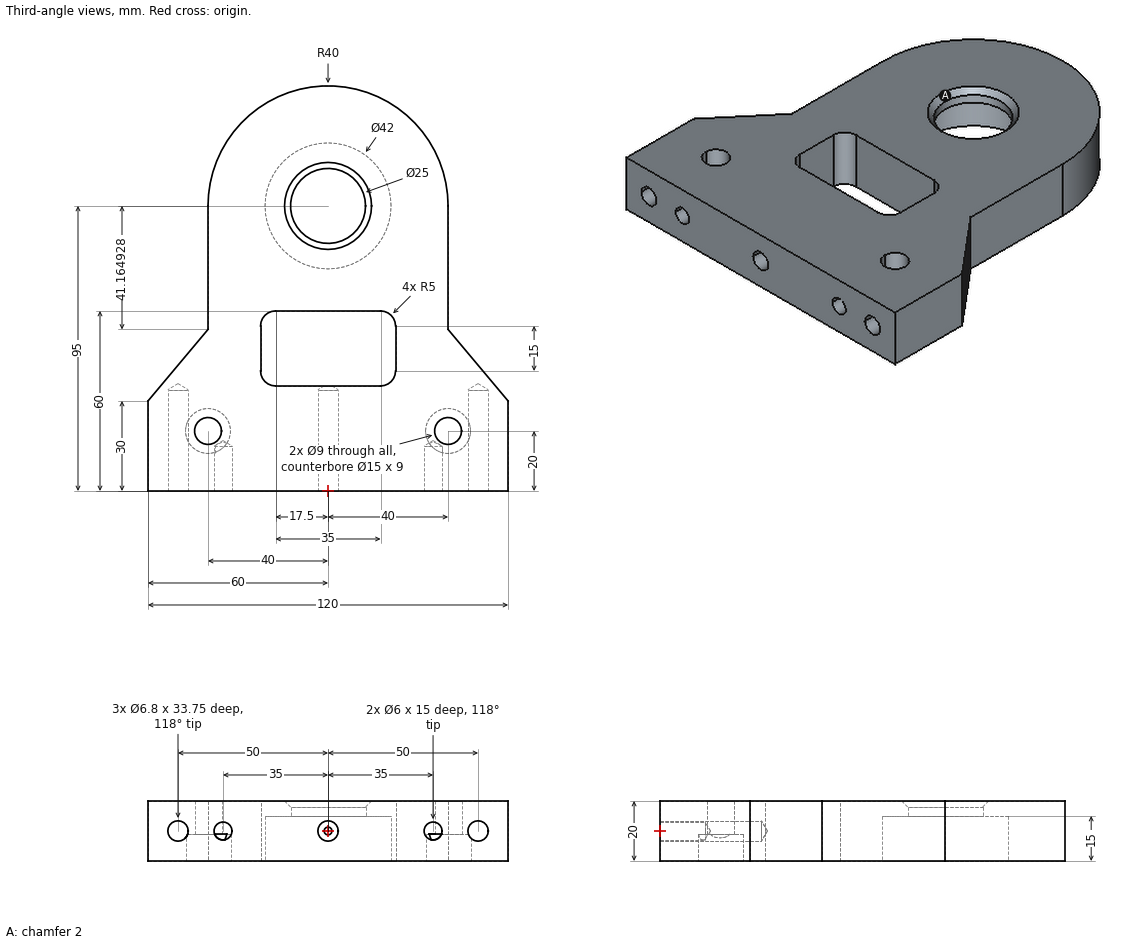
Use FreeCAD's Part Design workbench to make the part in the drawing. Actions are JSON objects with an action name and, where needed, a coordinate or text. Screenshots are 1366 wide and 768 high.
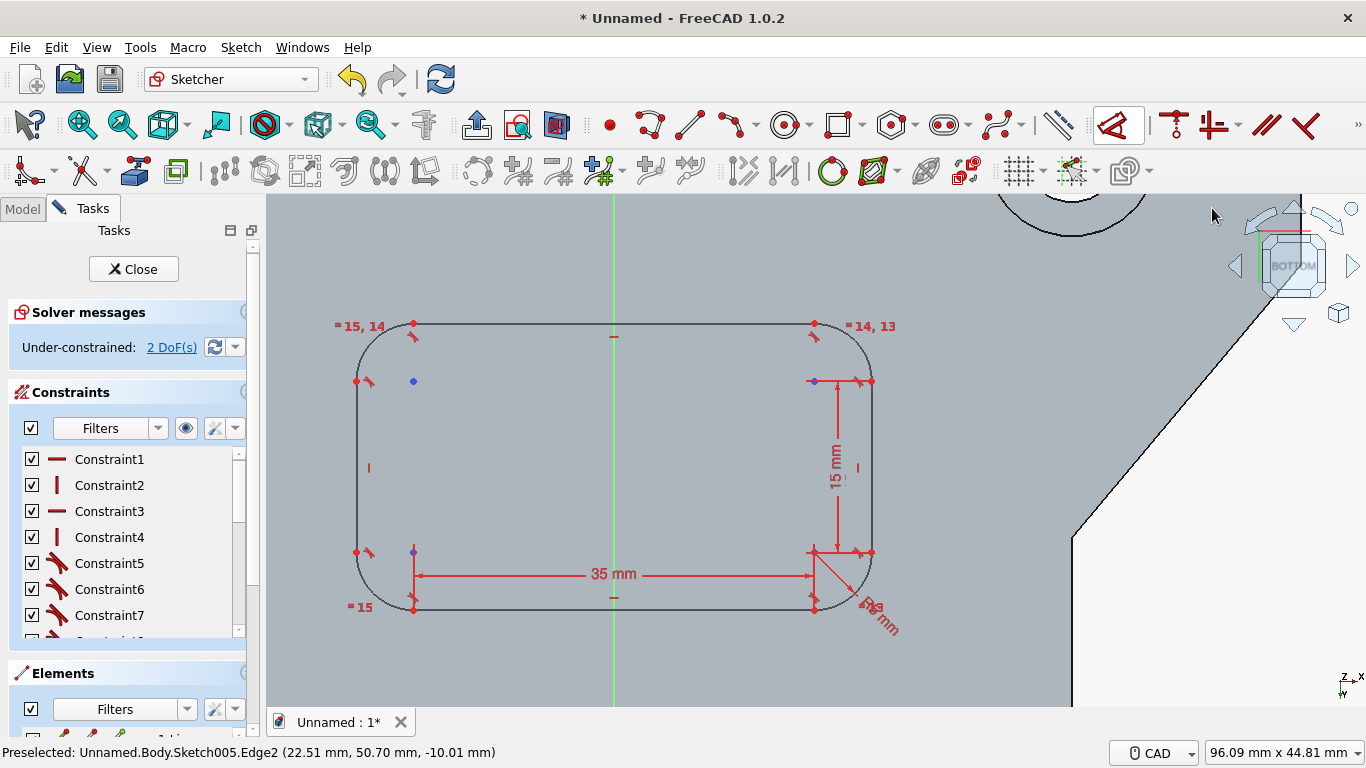
{"action": "left_click", "coordinate": [414, 610]}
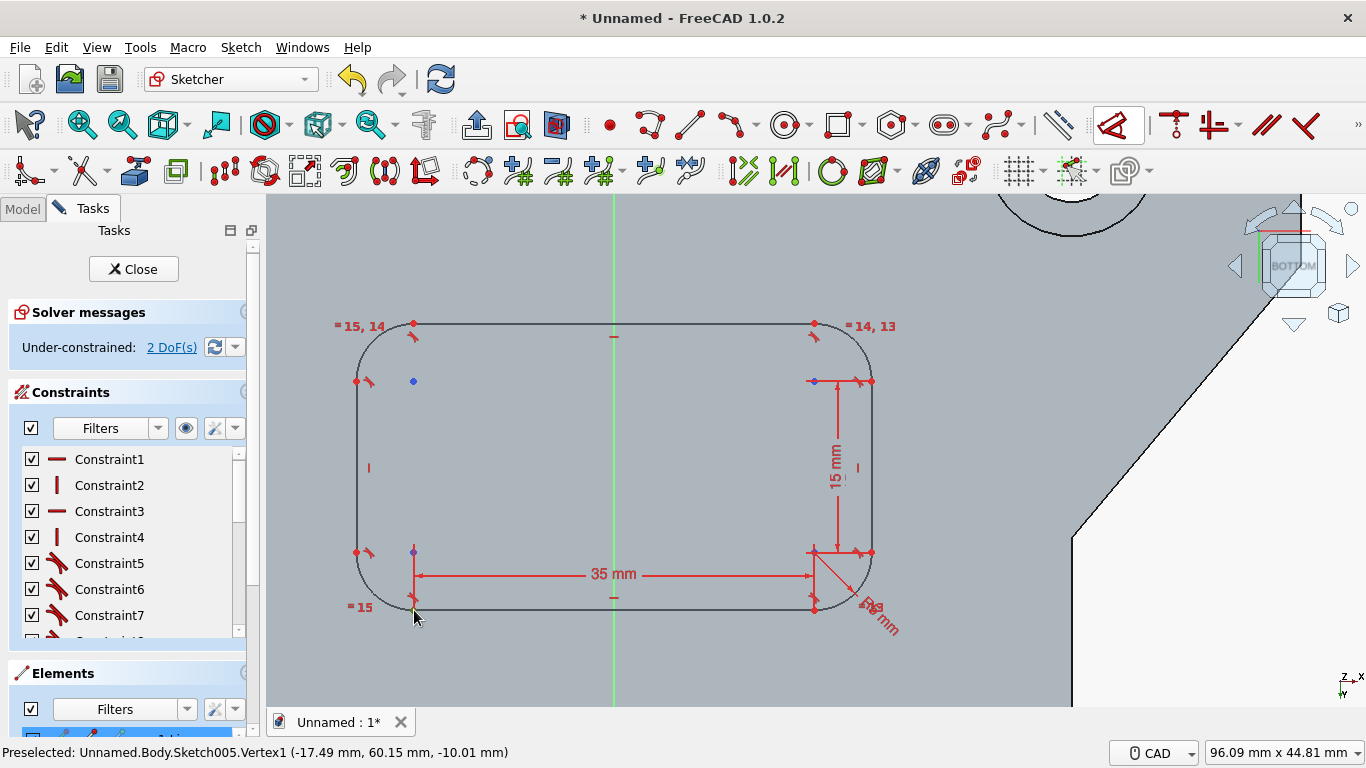
{"action": "left_click", "coordinate": [1138, 126]}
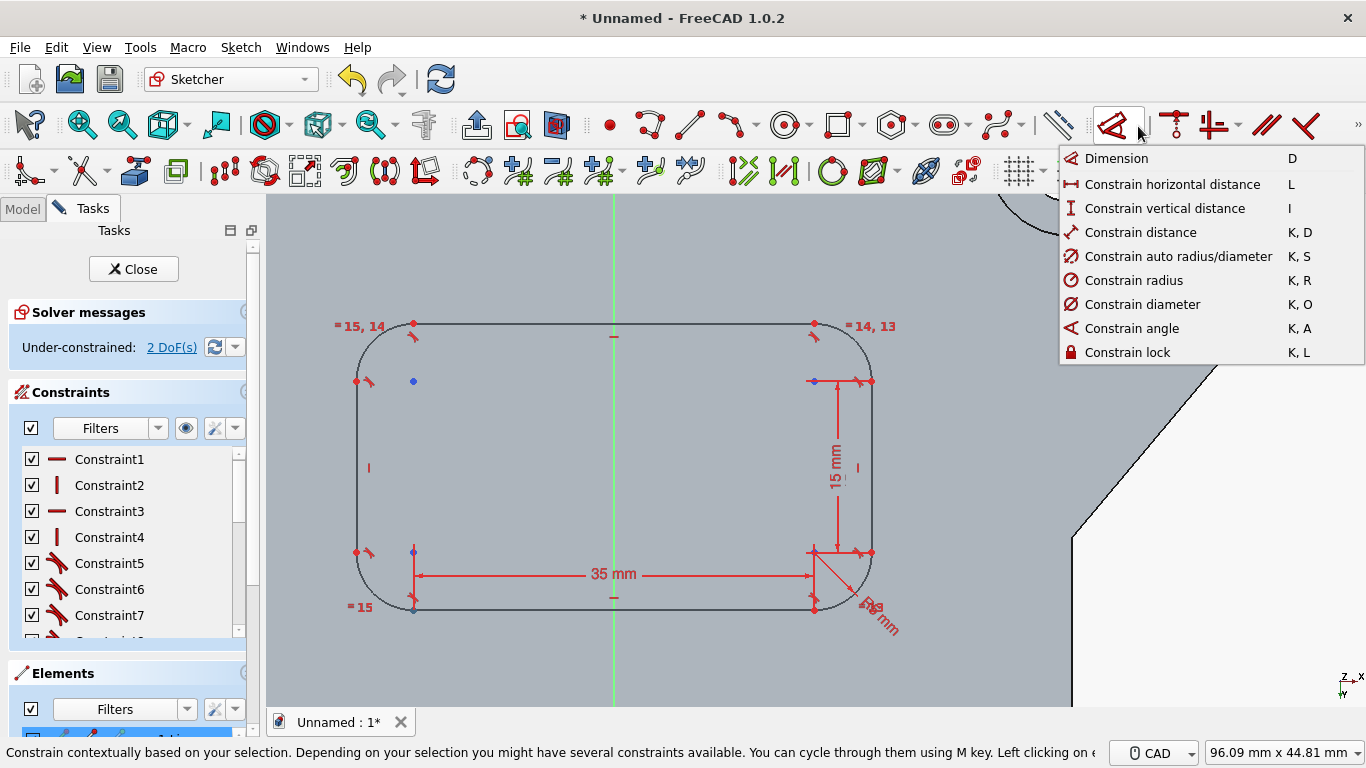
{"action": "left_click", "coordinate": [1212, 208]}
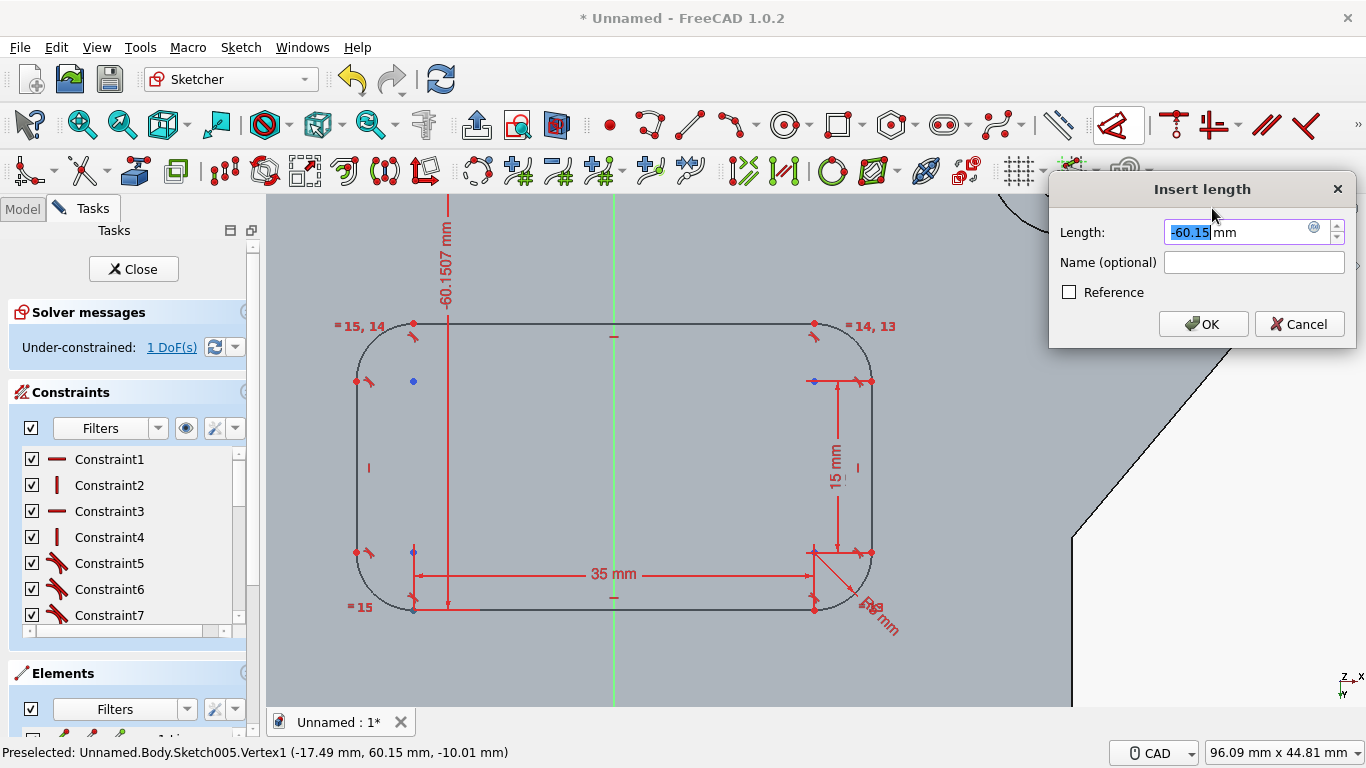
{"action": "type", "text": "-60"}
{"action": "key", "text": "Return"}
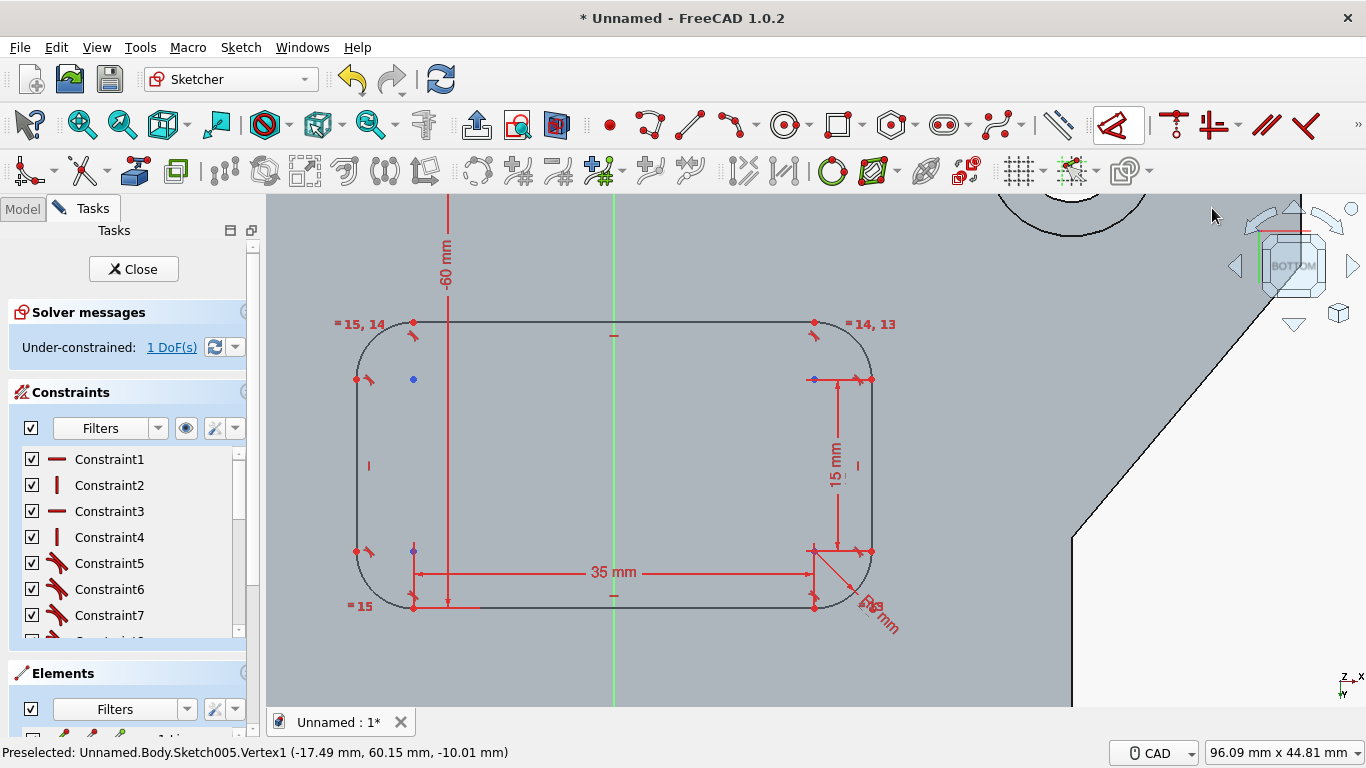
{"action": "left_click", "coordinate": [414, 608]}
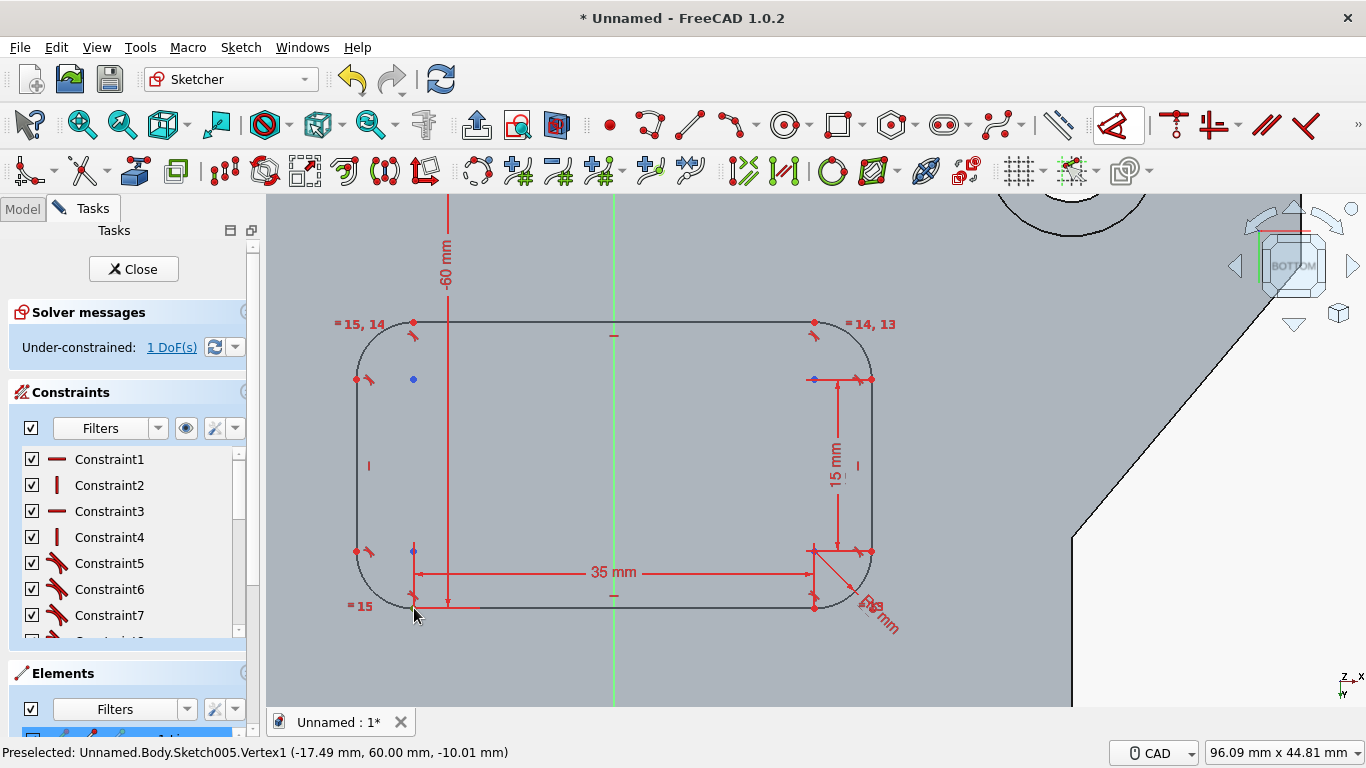
{"action": "key", "text": "l"}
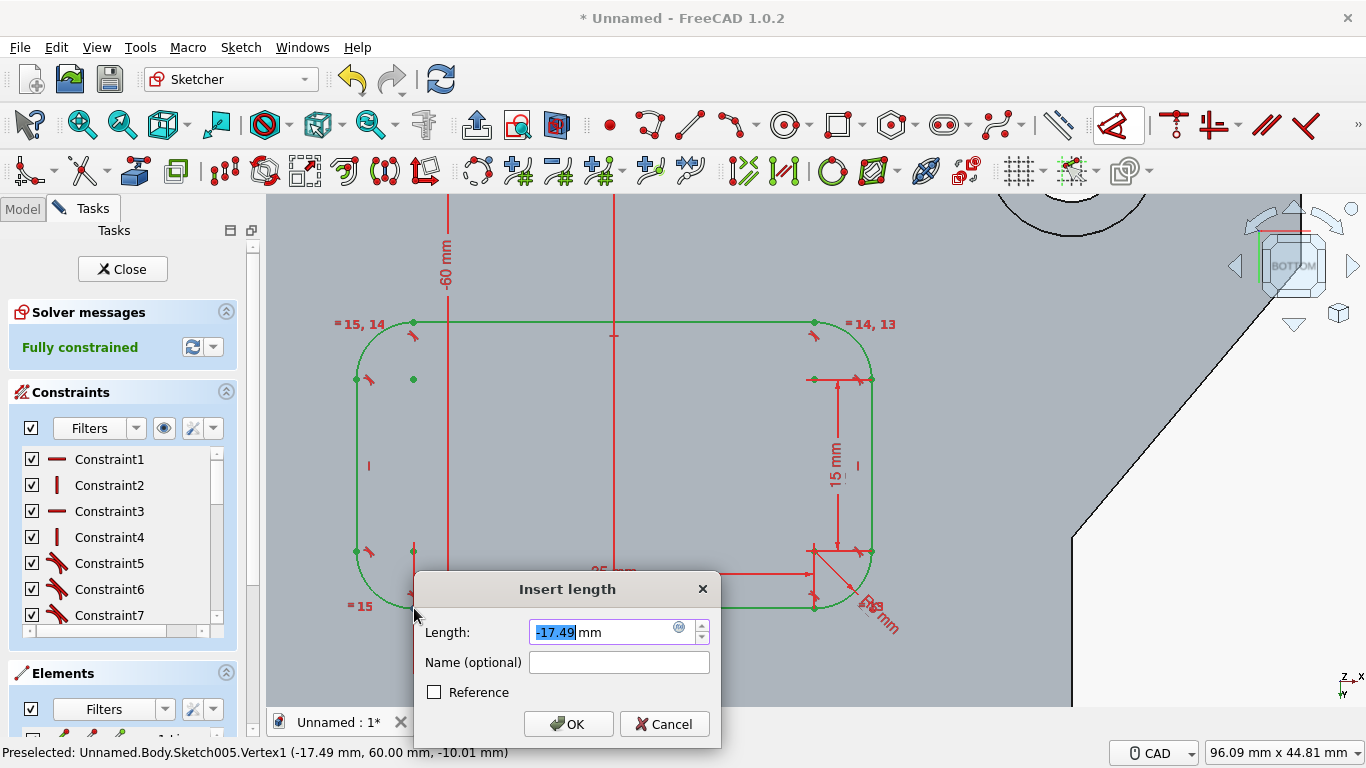
{"action": "type", "text": "-17.5"}
{"action": "key", "text": "Return"}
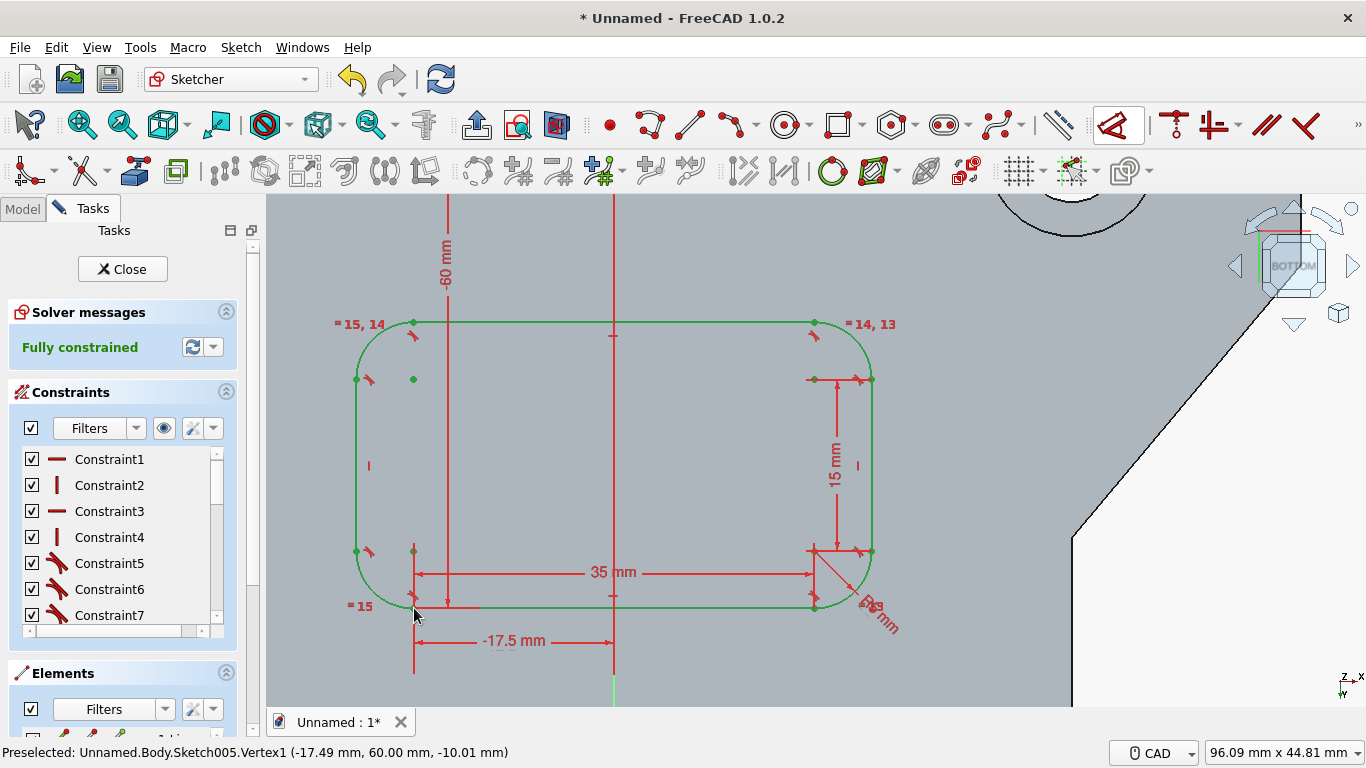
{"action": "left_click", "coordinate": [123, 269]}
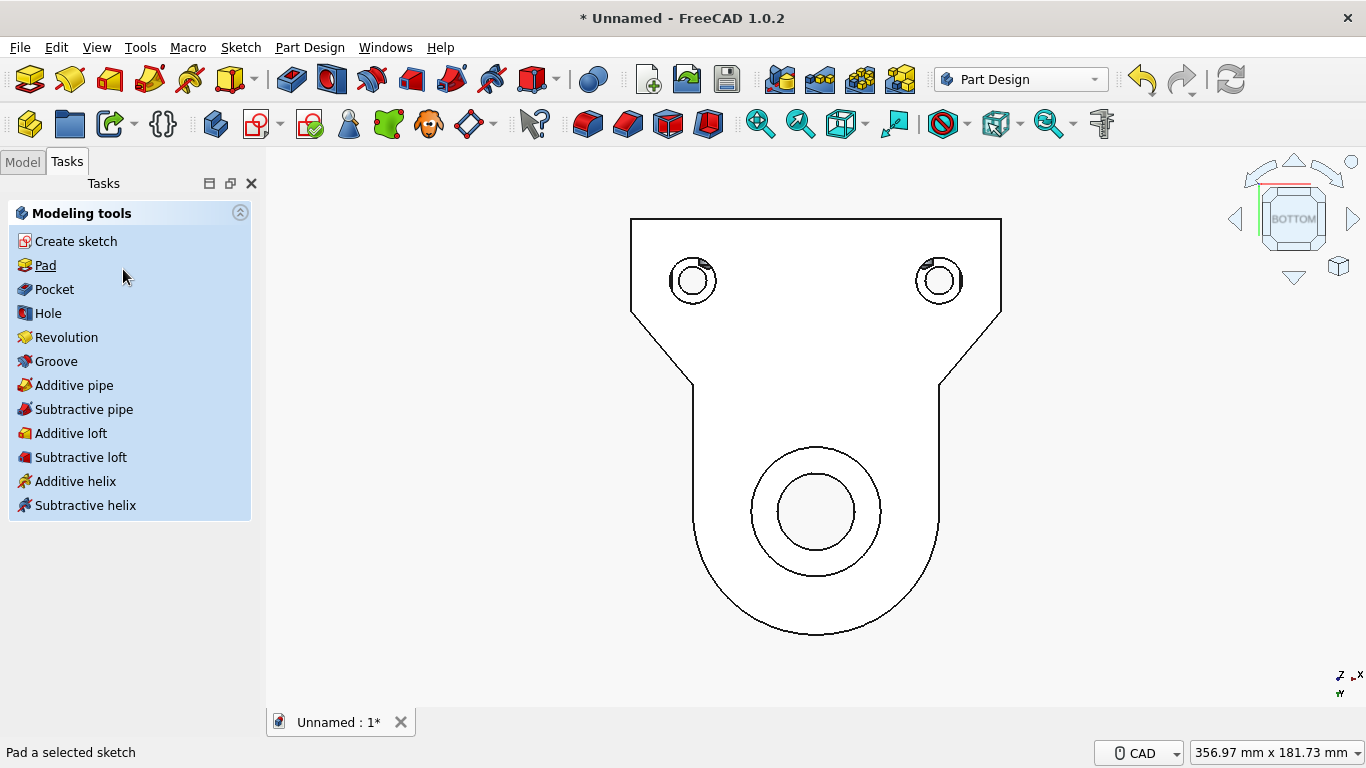
{"action": "left_click", "coordinate": [292, 80]}